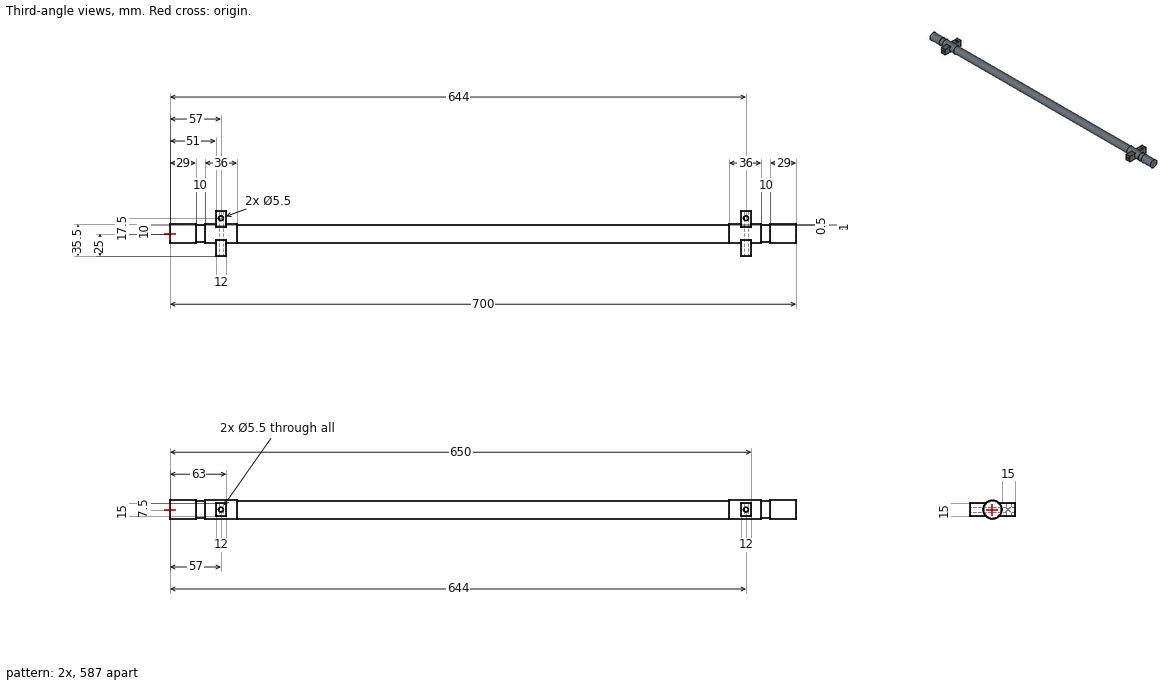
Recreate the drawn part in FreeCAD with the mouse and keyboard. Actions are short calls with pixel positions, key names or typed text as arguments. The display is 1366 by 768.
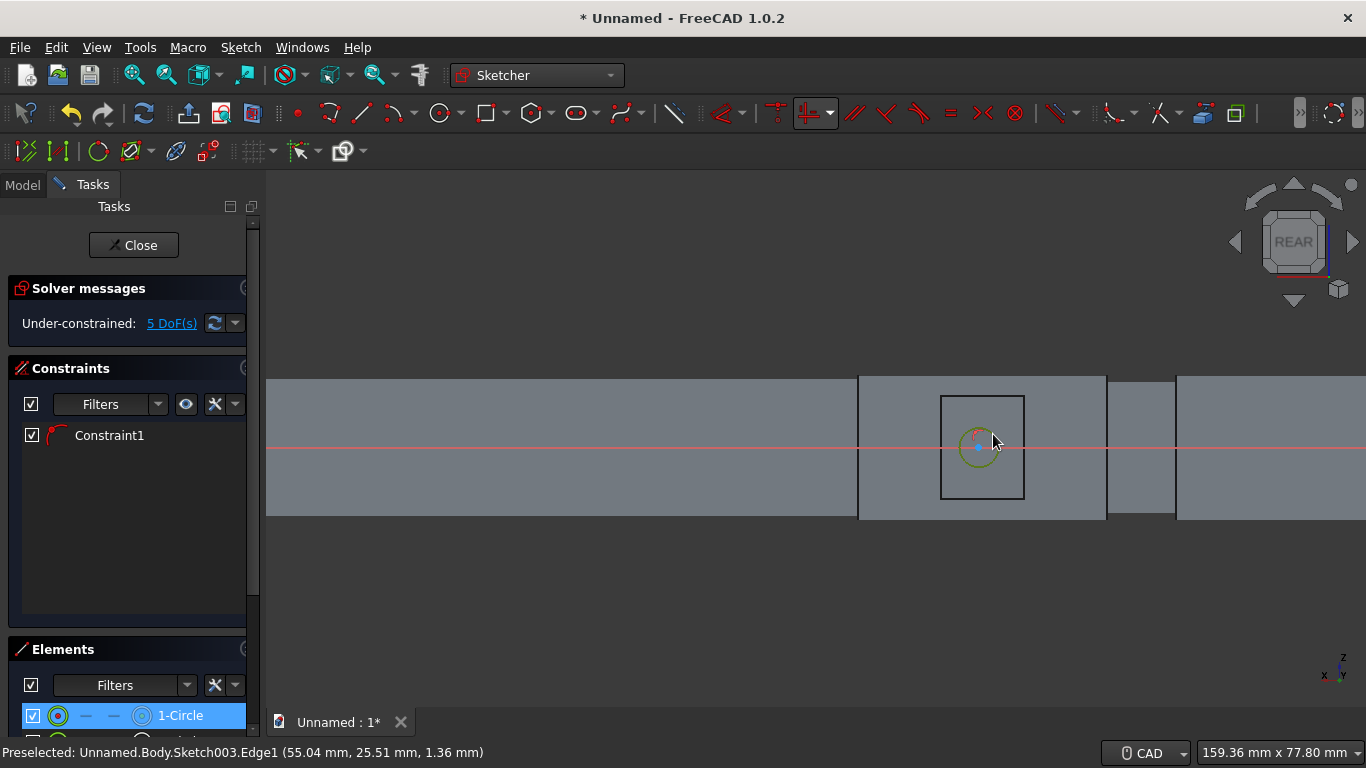
scroll(998, 437, down, 10)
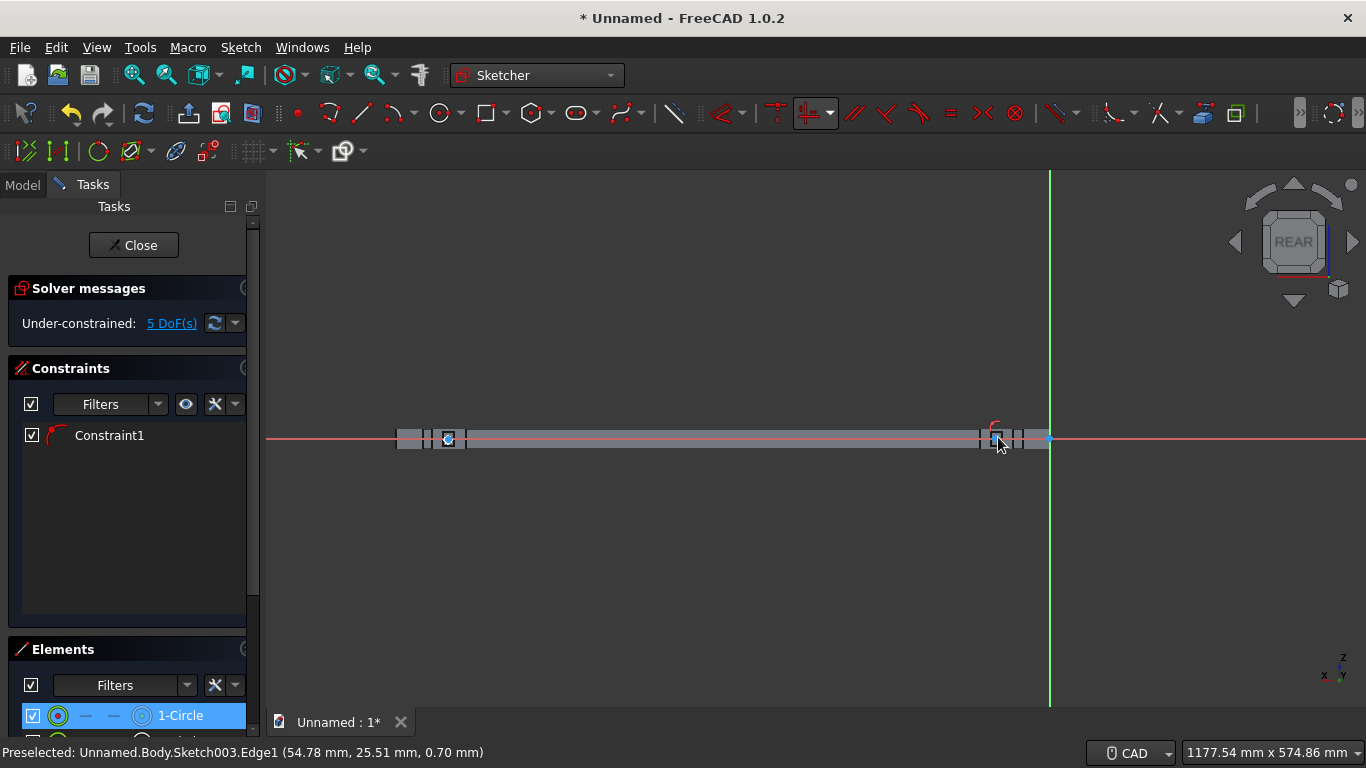
scroll(451, 437, up, 12)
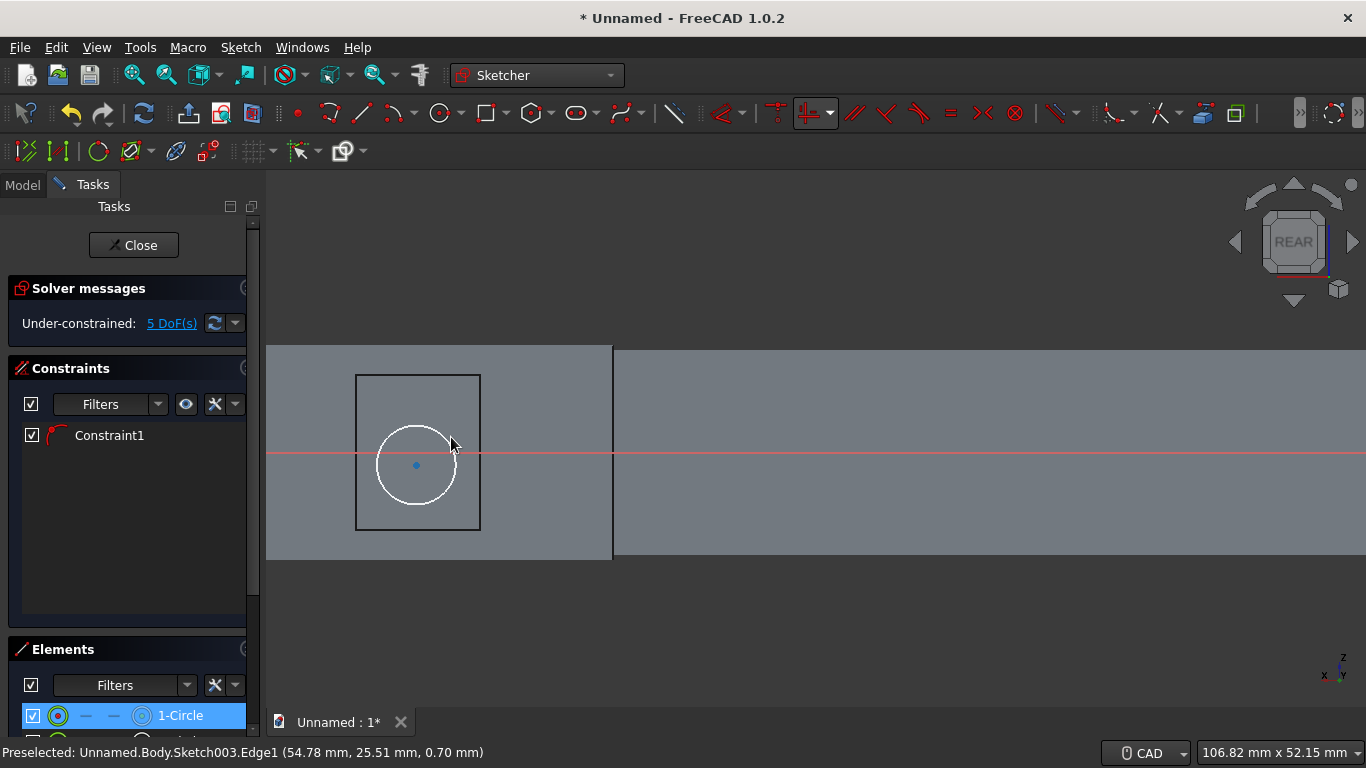
click(444, 437)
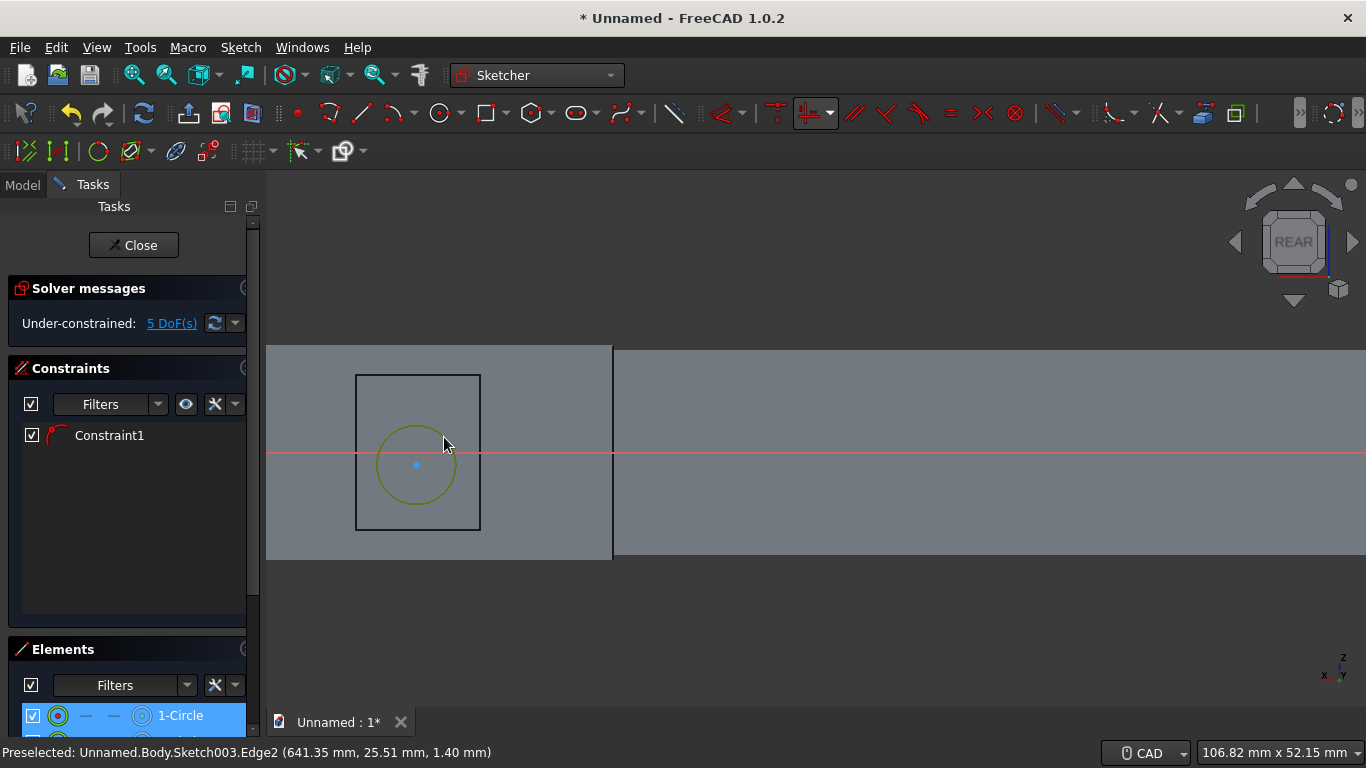
click(952, 114)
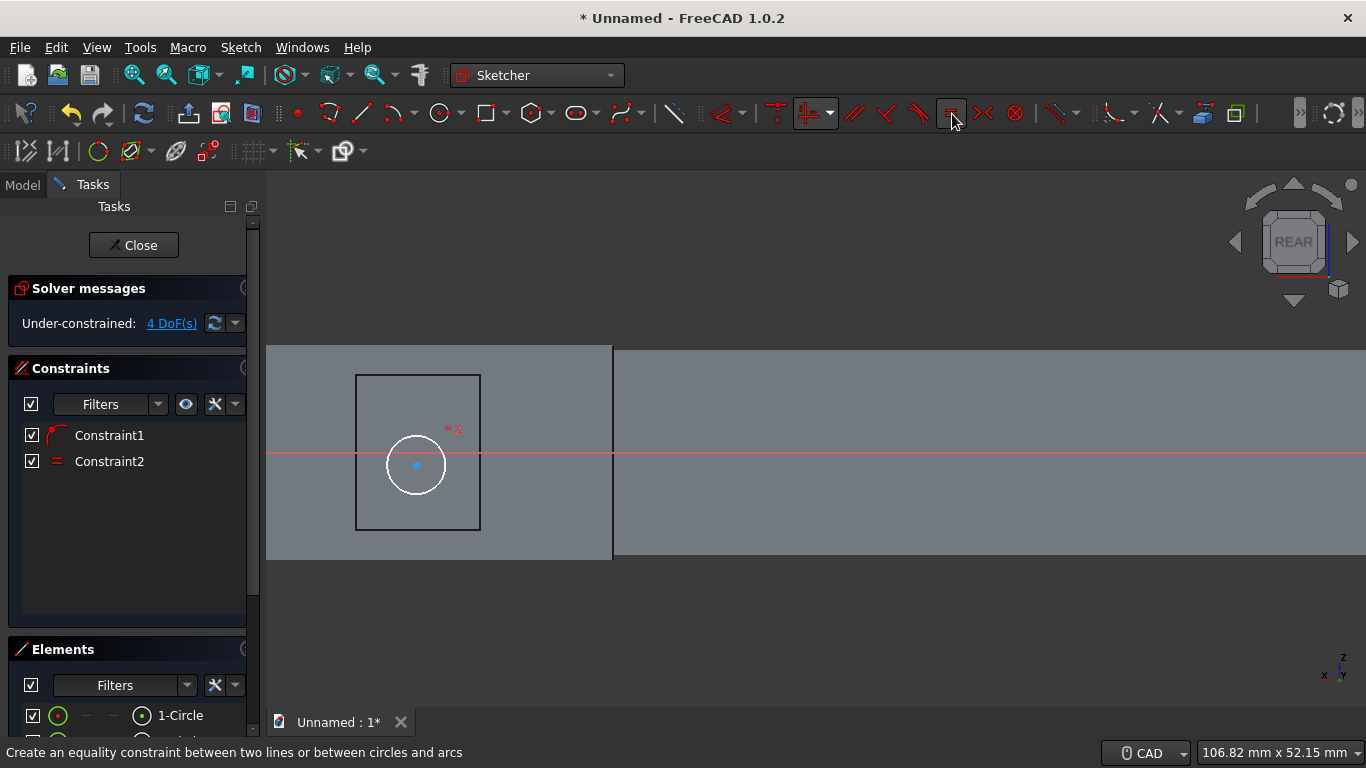
scroll(451, 437, down, 12)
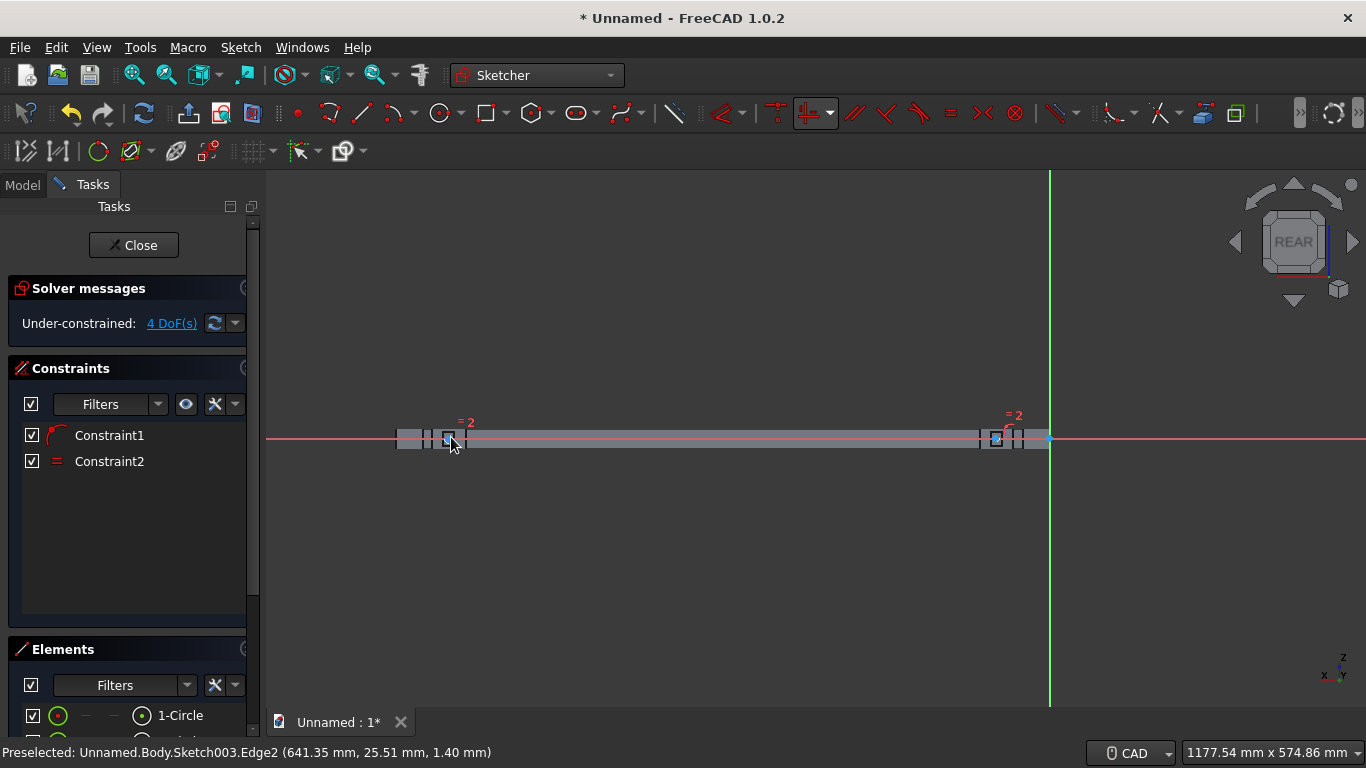
click(448, 440)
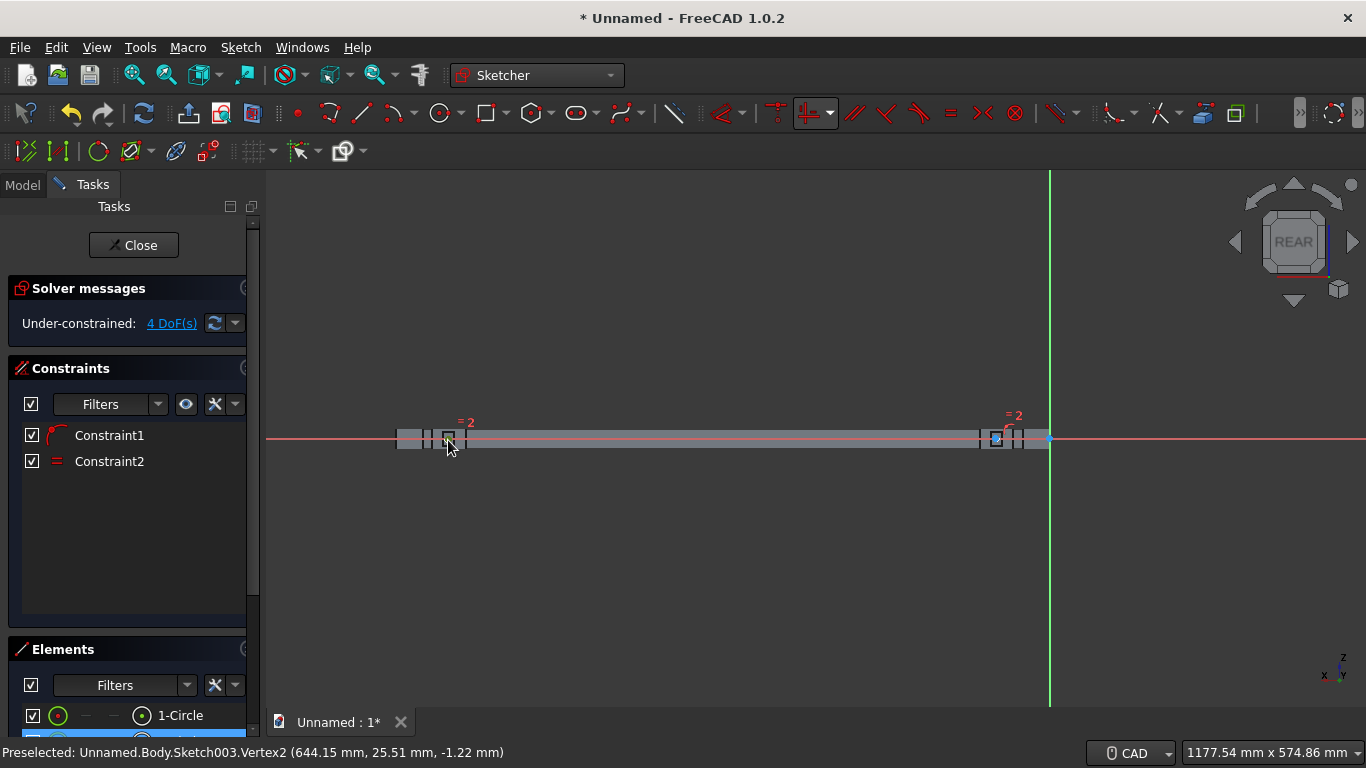
click(359, 439)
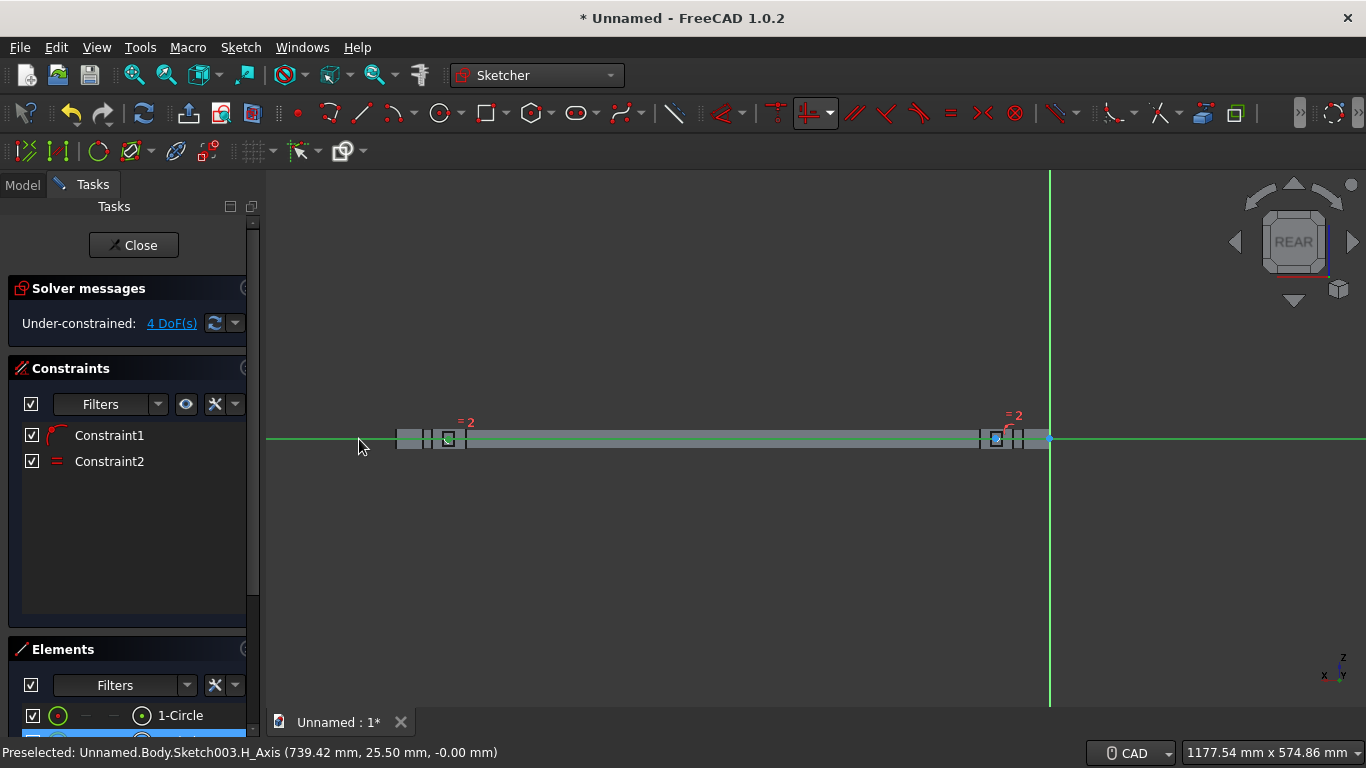
click(776, 114)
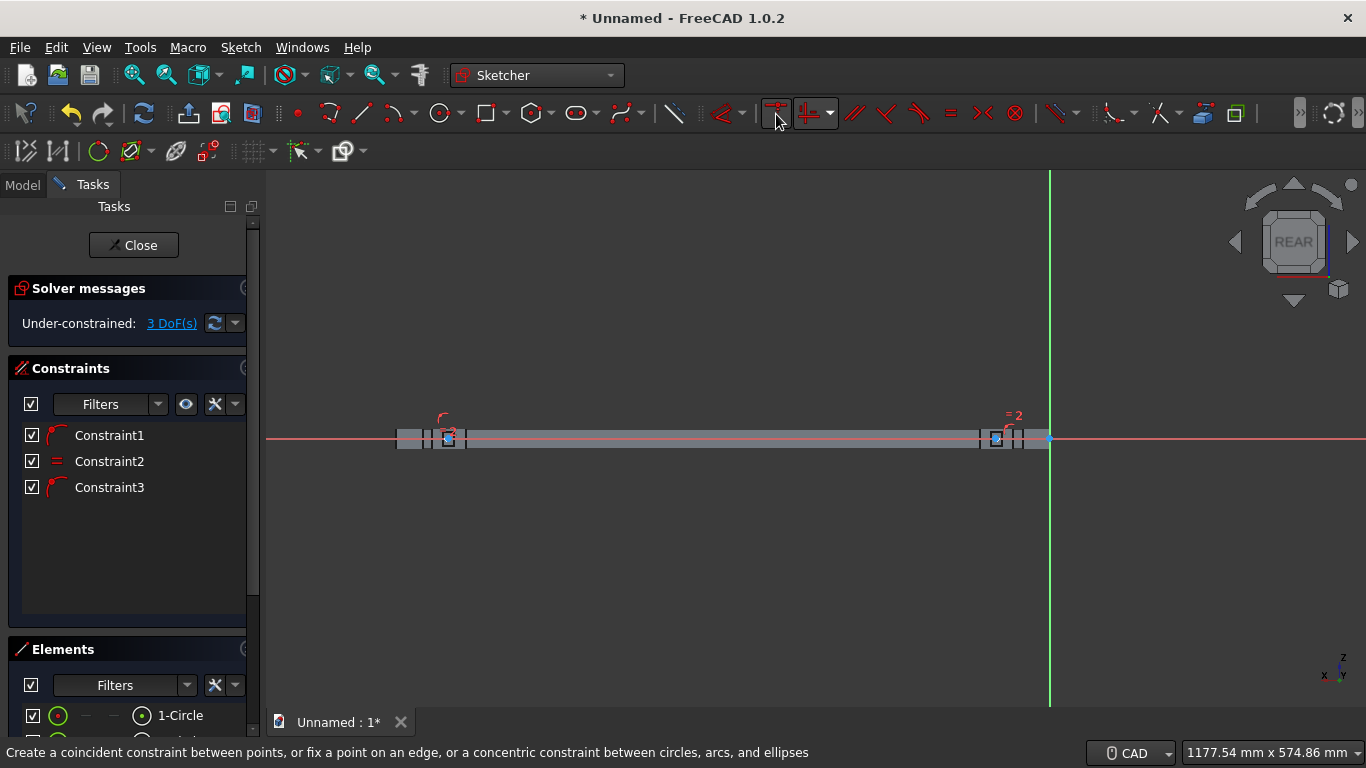
click(722, 114)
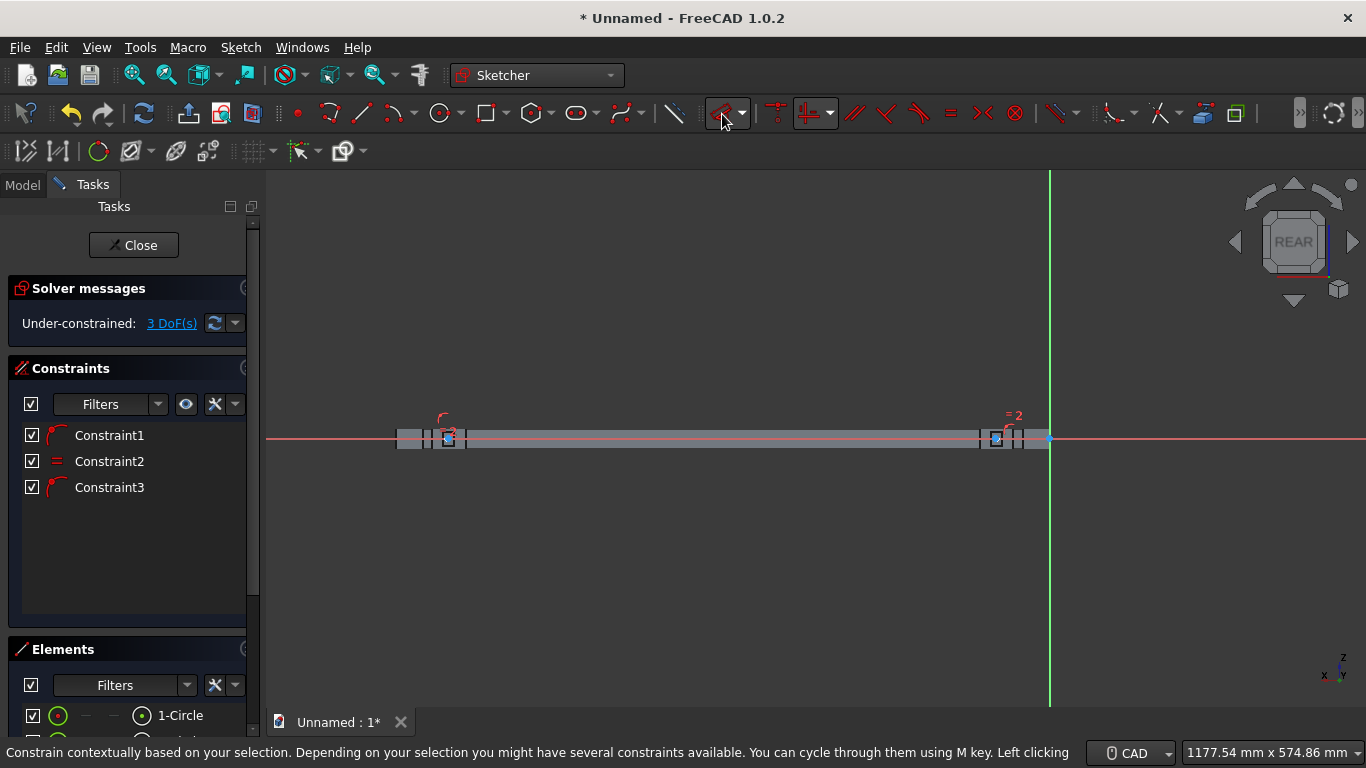
scroll(994, 437, up, 11)